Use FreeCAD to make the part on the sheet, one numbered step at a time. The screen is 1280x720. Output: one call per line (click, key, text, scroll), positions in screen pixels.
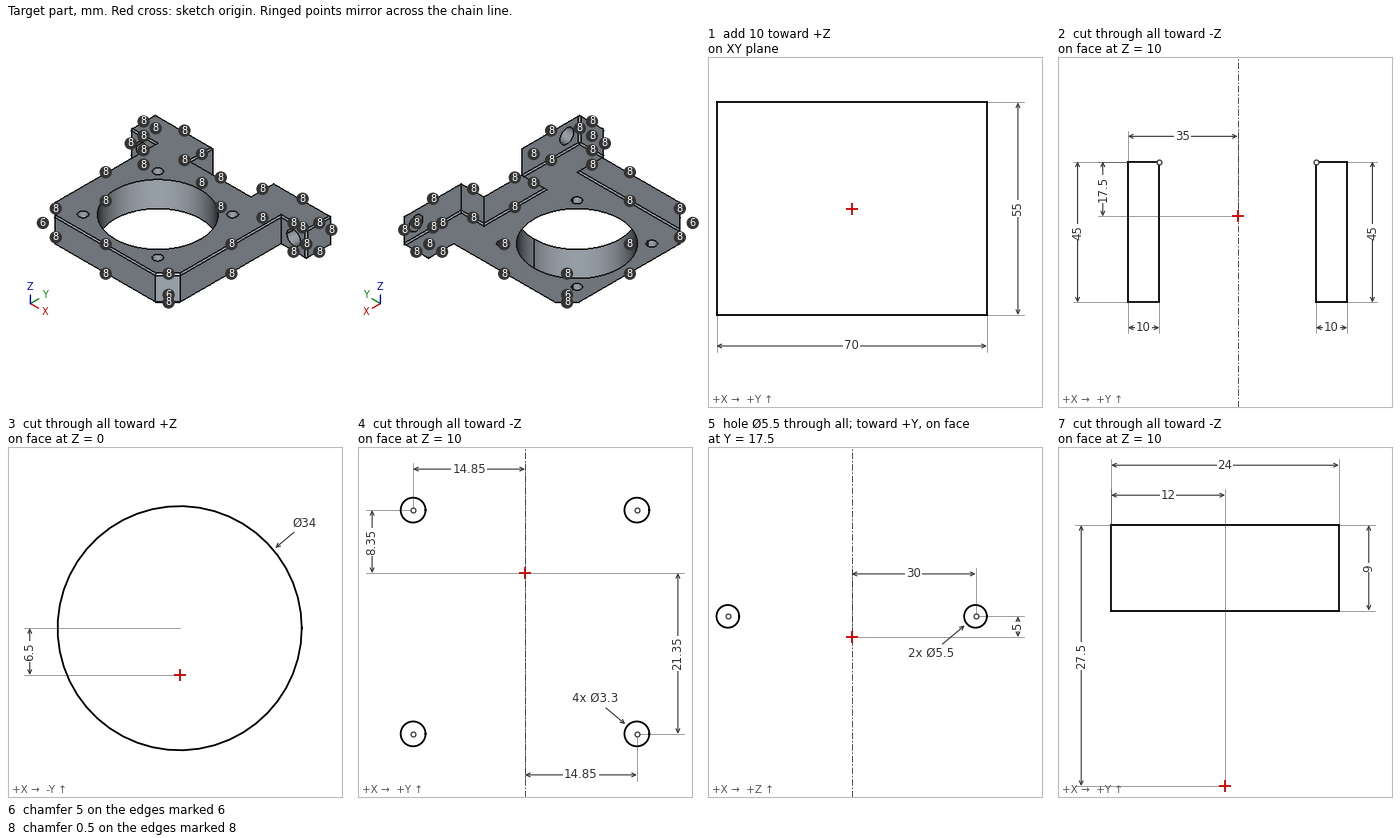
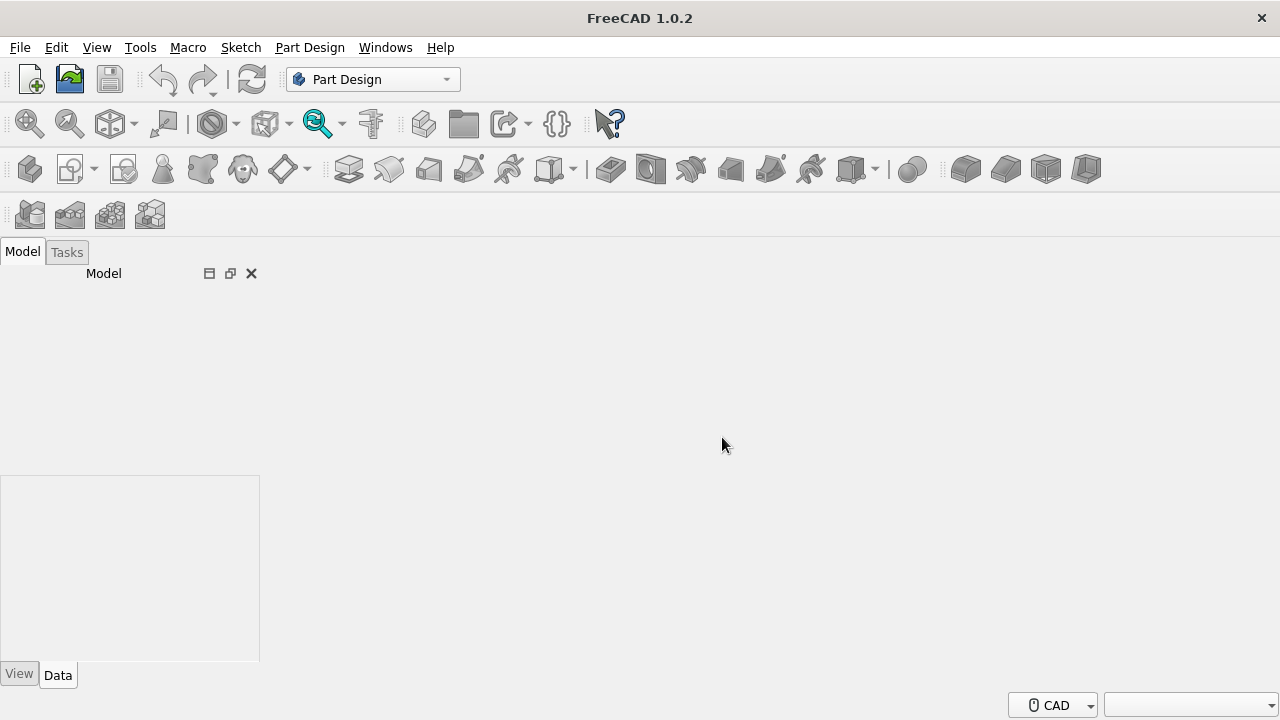
key(ctrl+n)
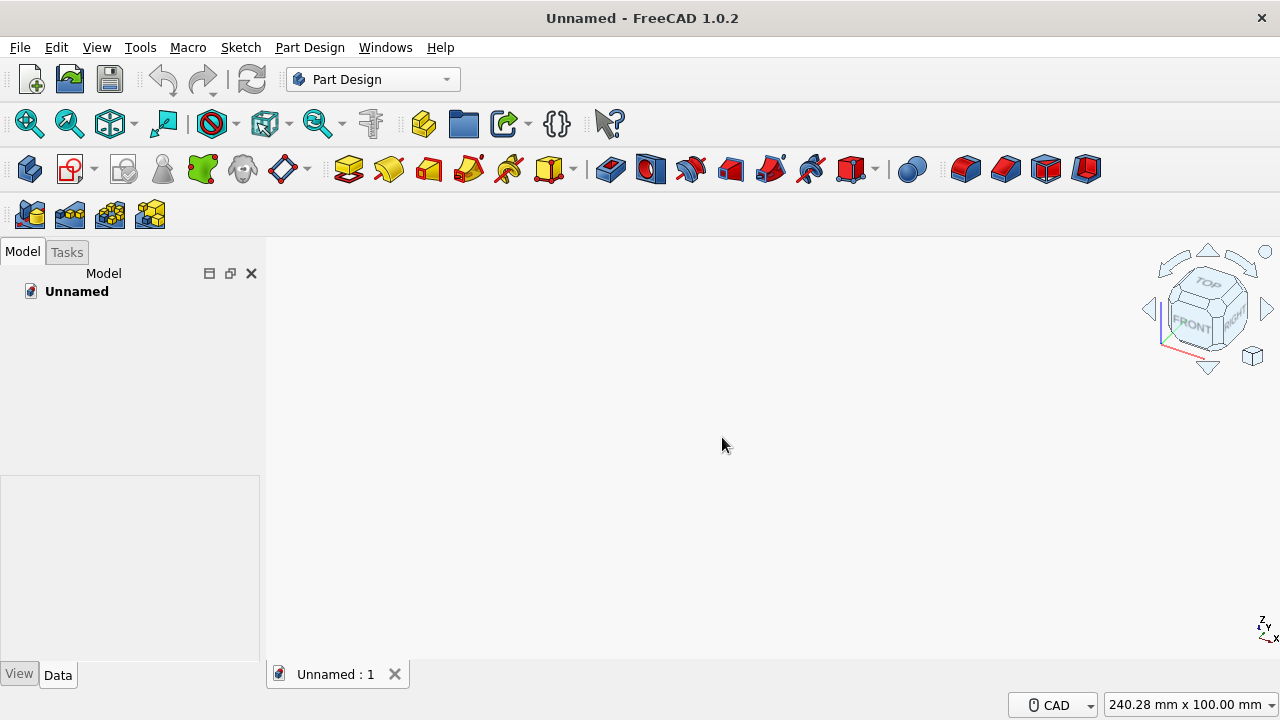
click(70, 170)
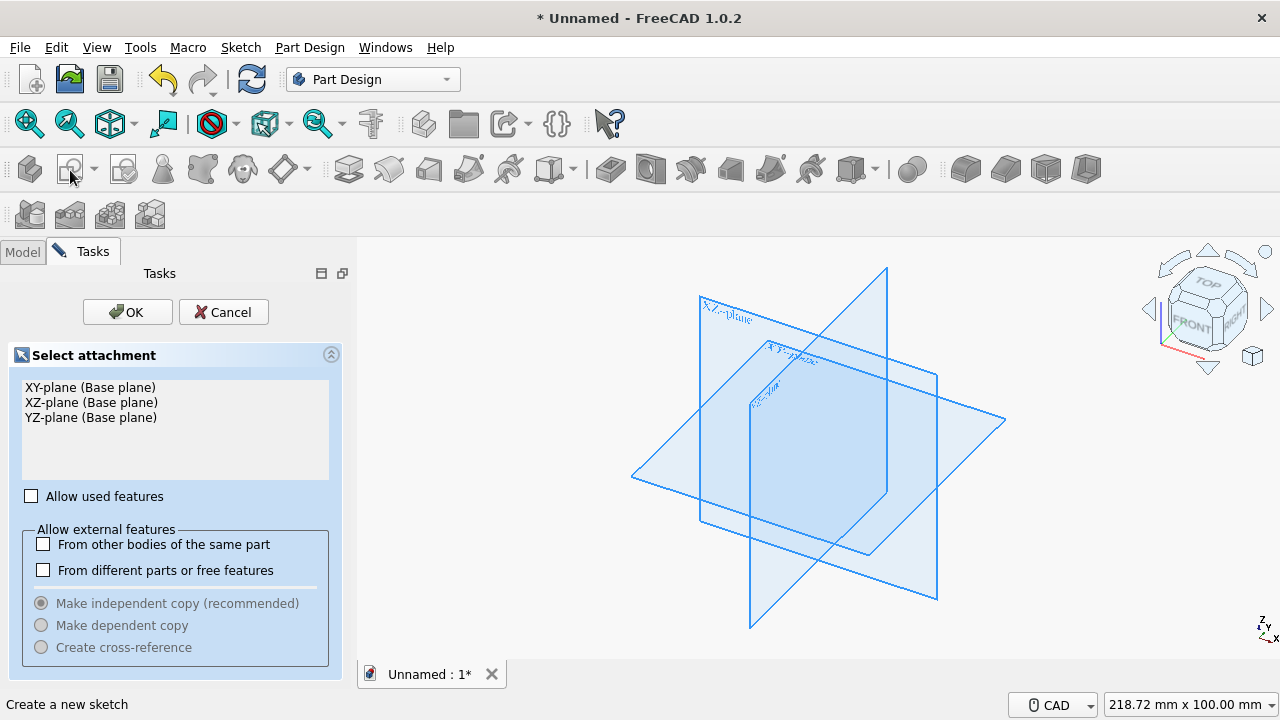
click(82, 388)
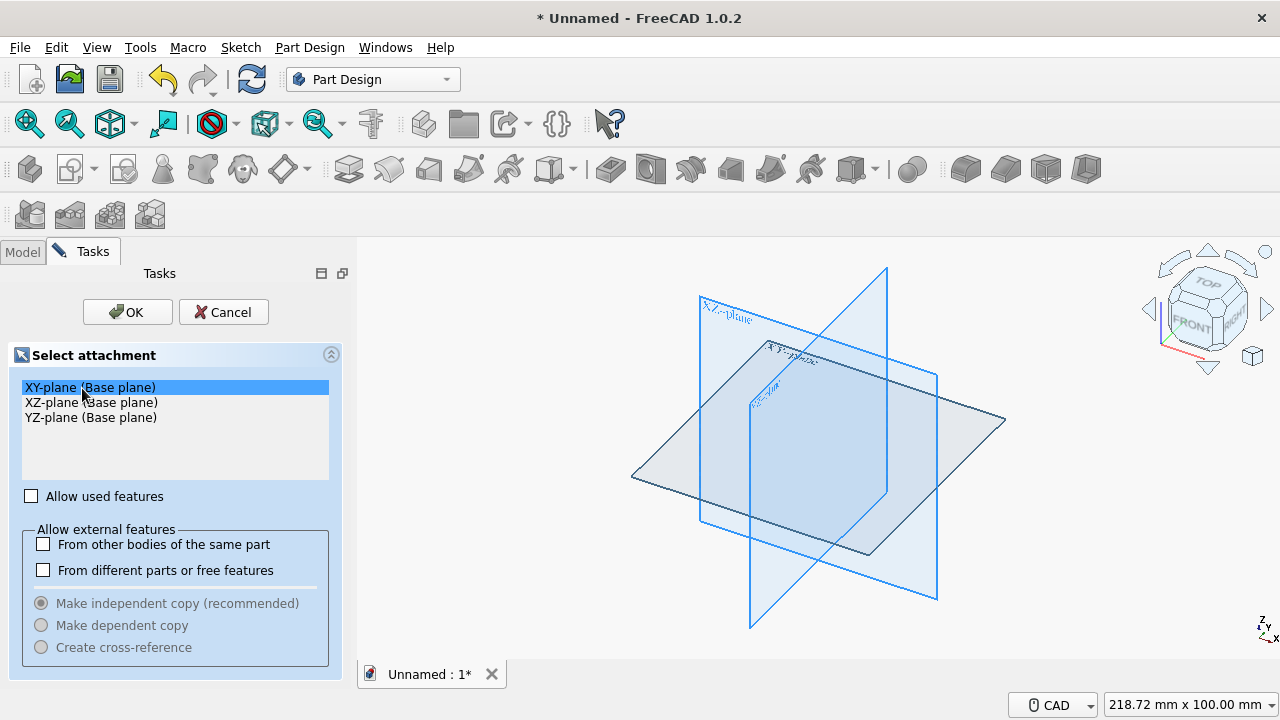
click(128, 312)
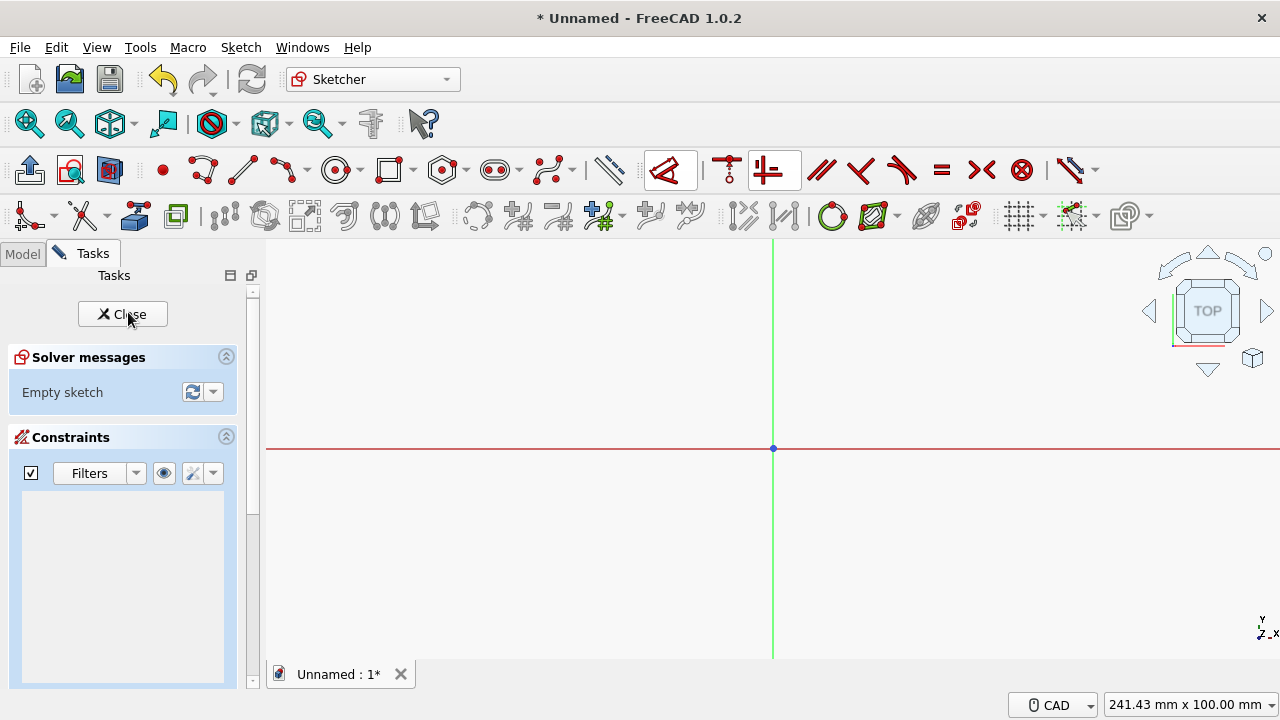
key(g)
key(v)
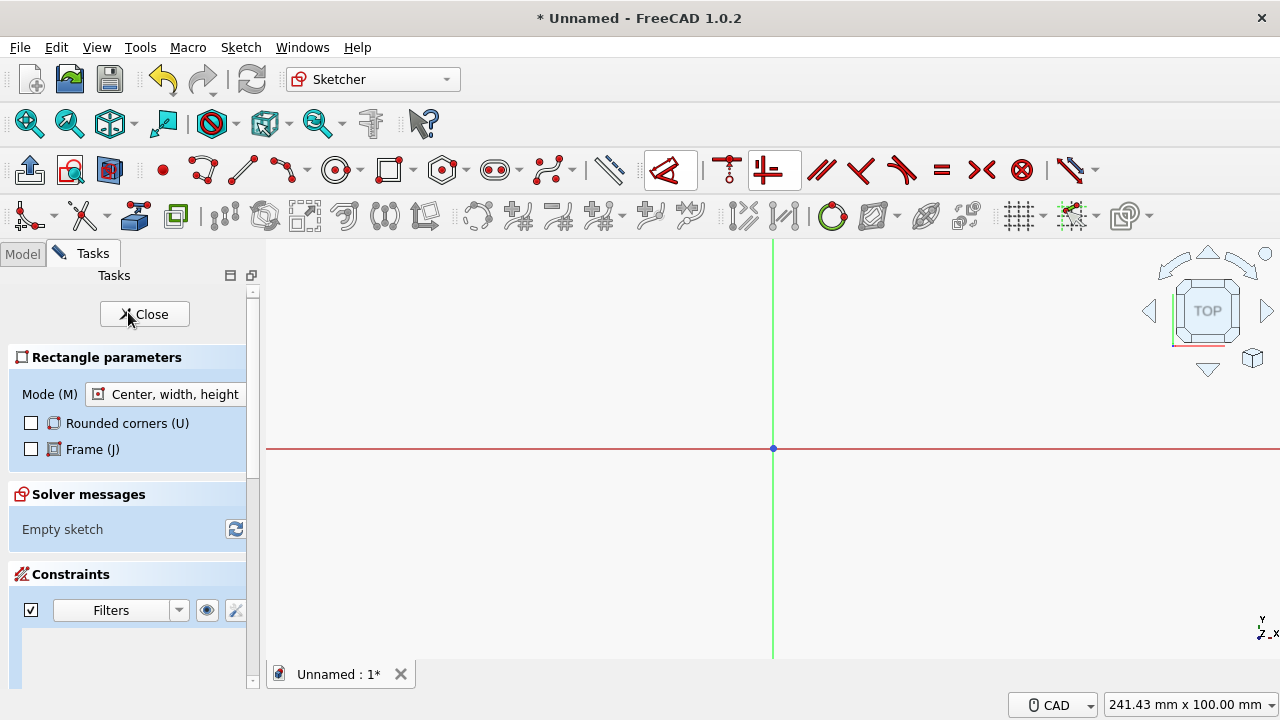
click(773, 449)
move(920, 334)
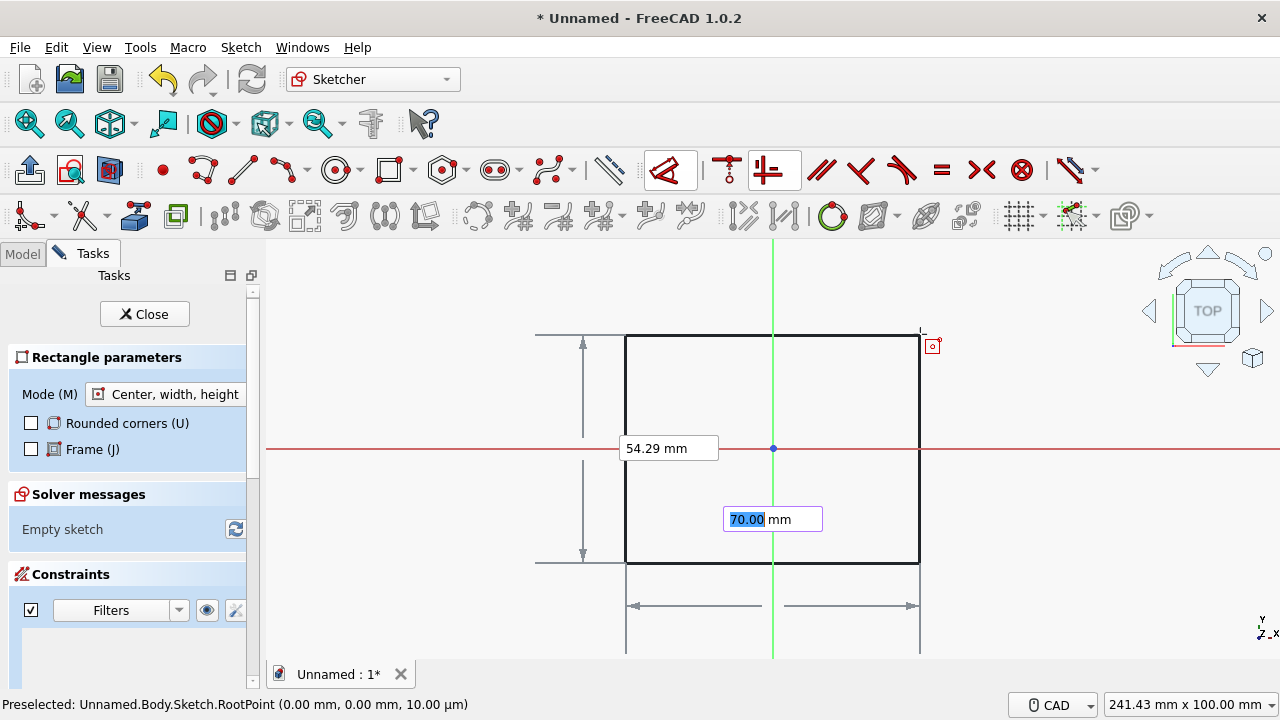
text(70)
key(Tab)
text(55)
key(Return)
key(Escape)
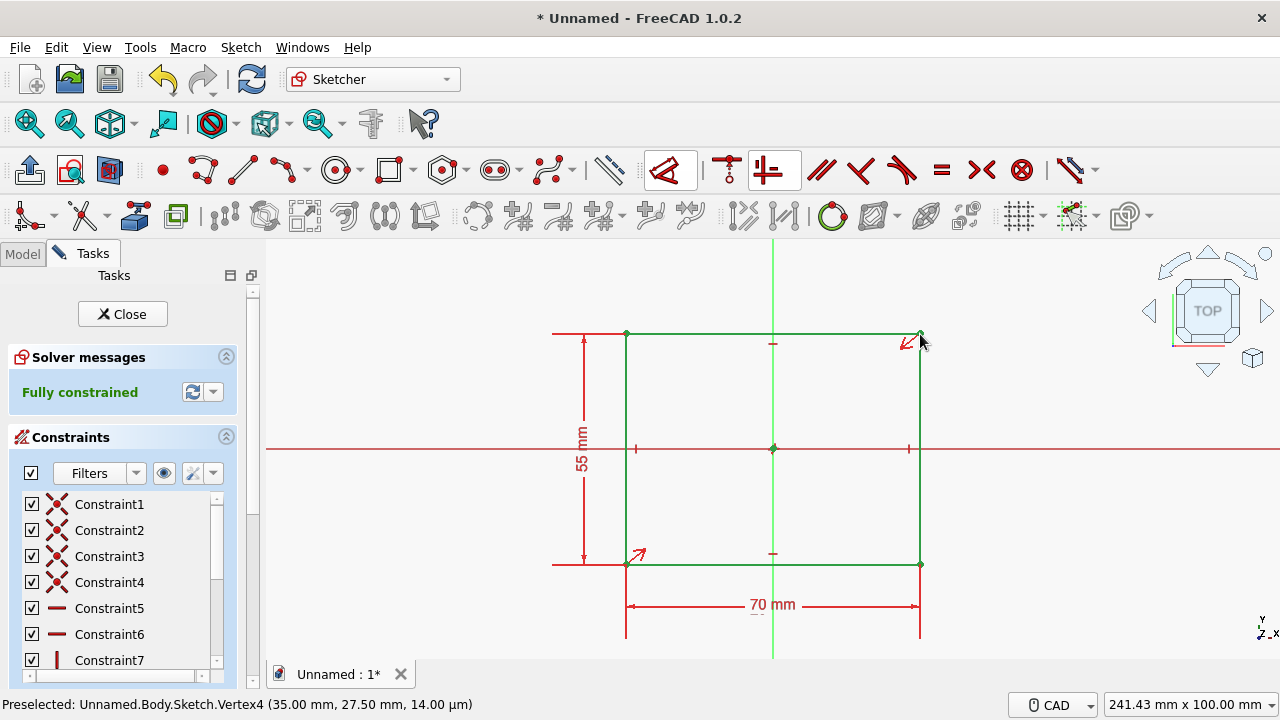
click(123, 314)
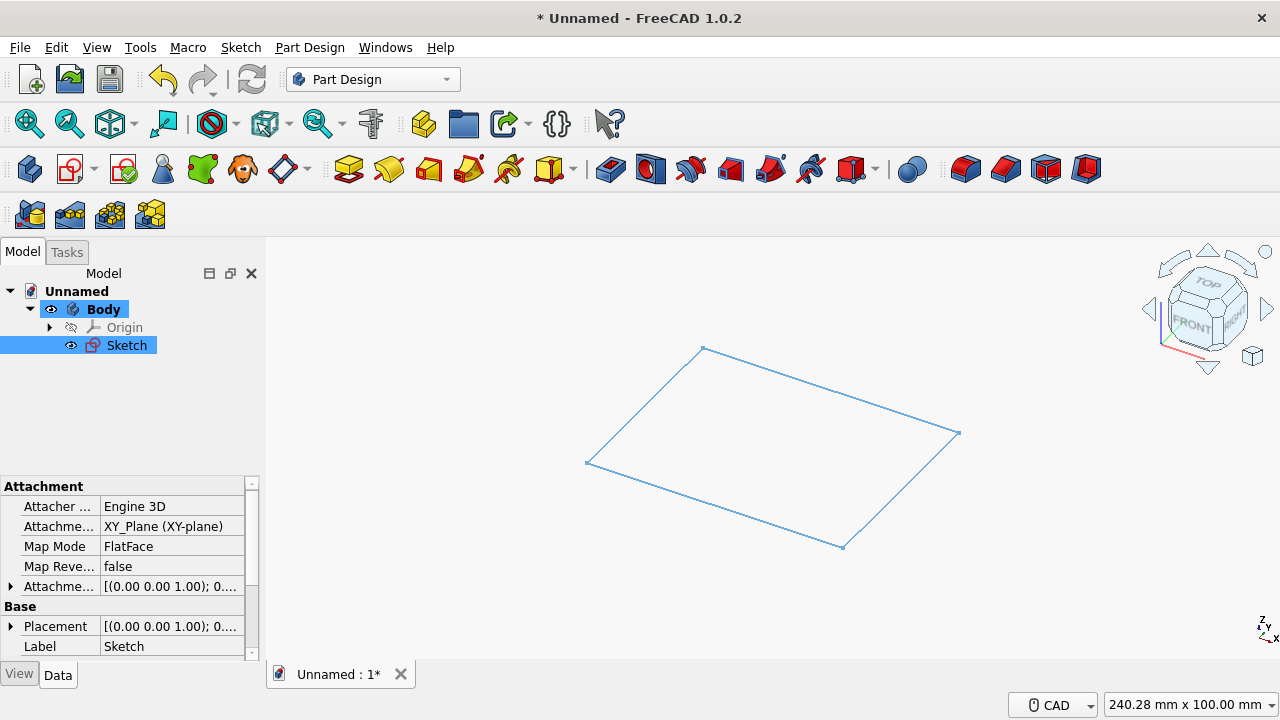
click(350, 170)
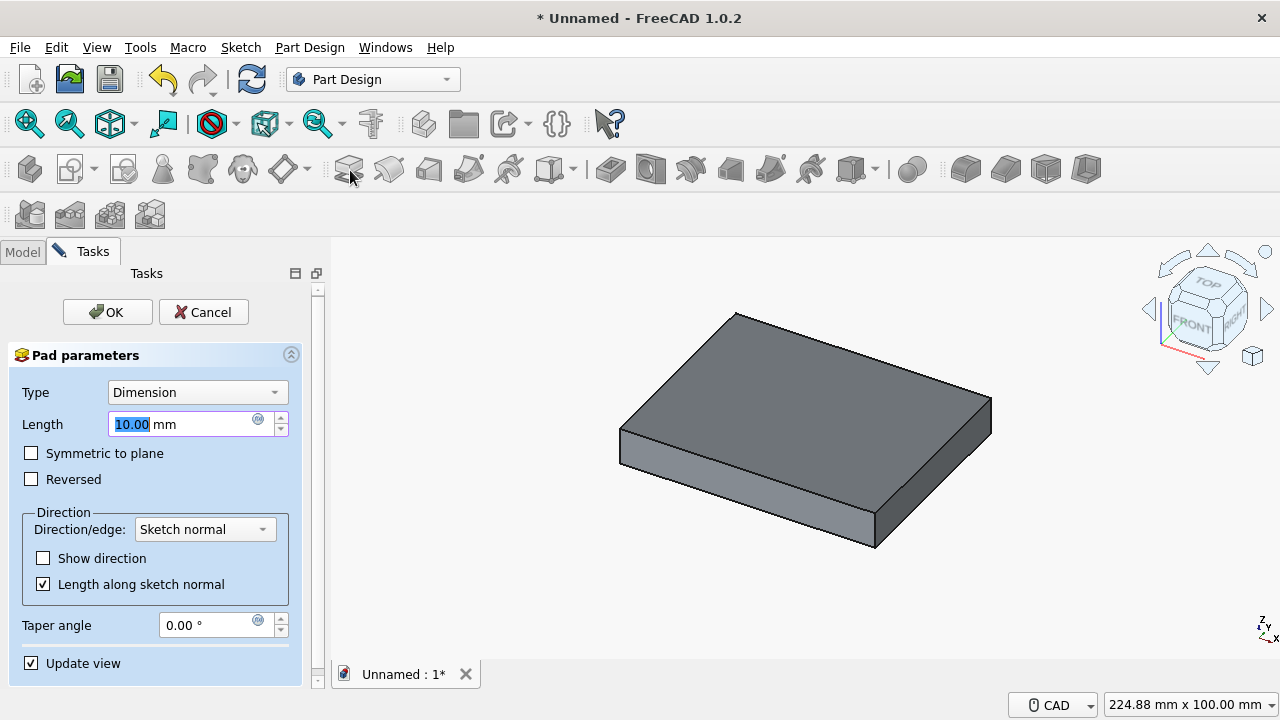
text(10)
key(Tab)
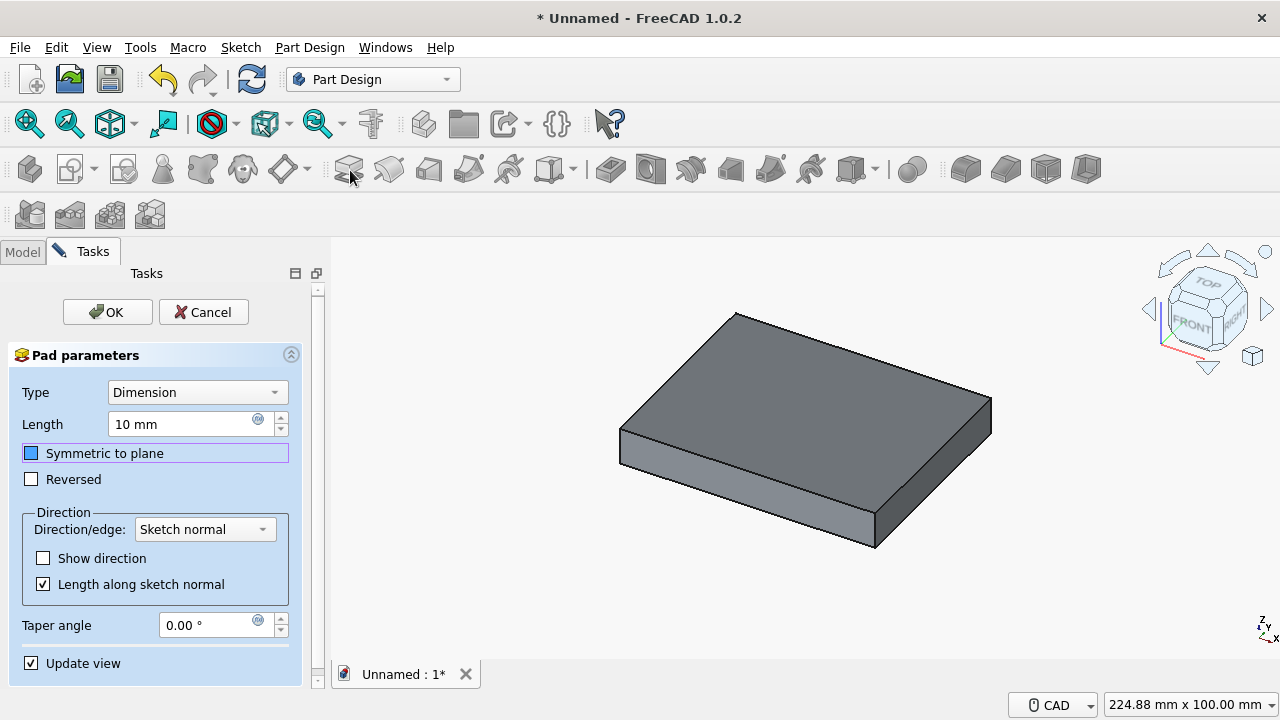
click(108, 312)